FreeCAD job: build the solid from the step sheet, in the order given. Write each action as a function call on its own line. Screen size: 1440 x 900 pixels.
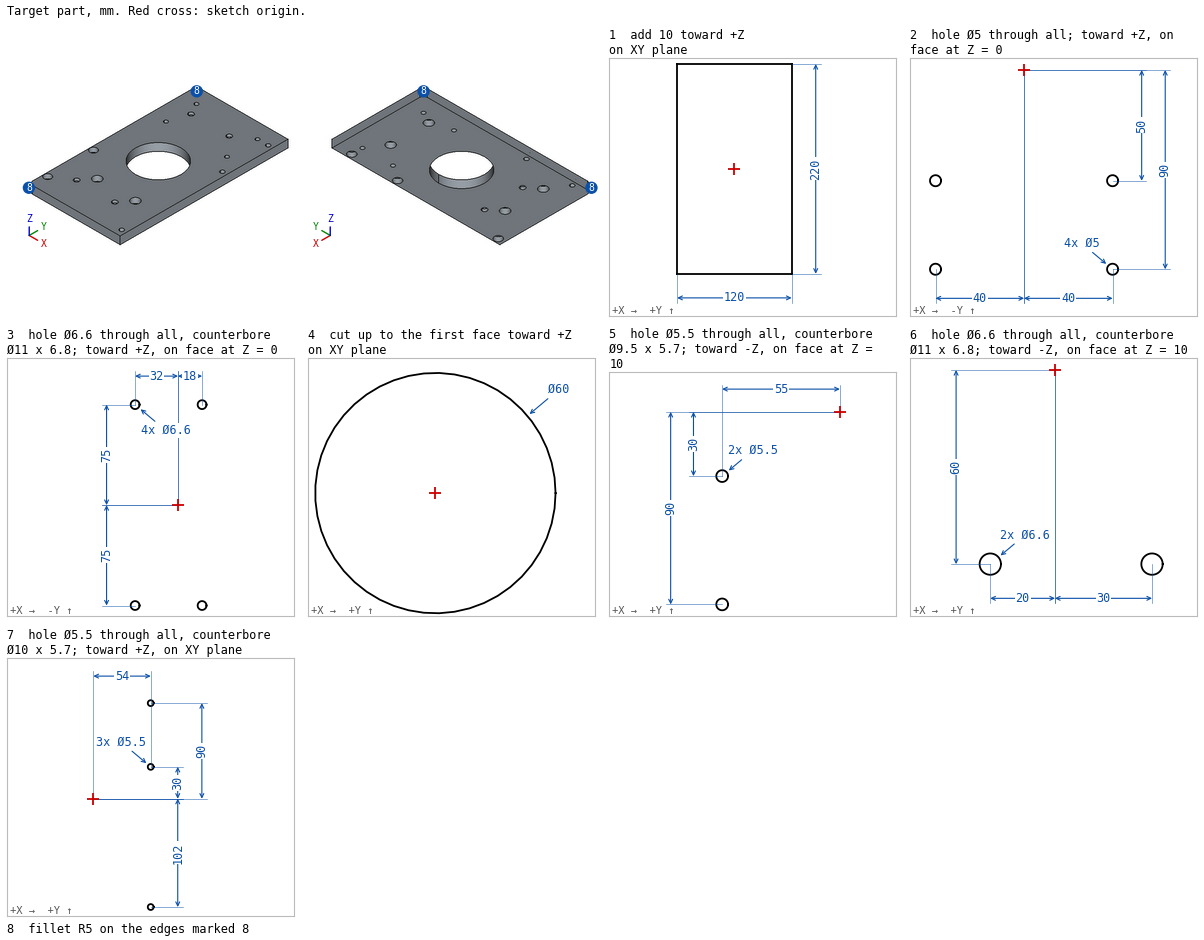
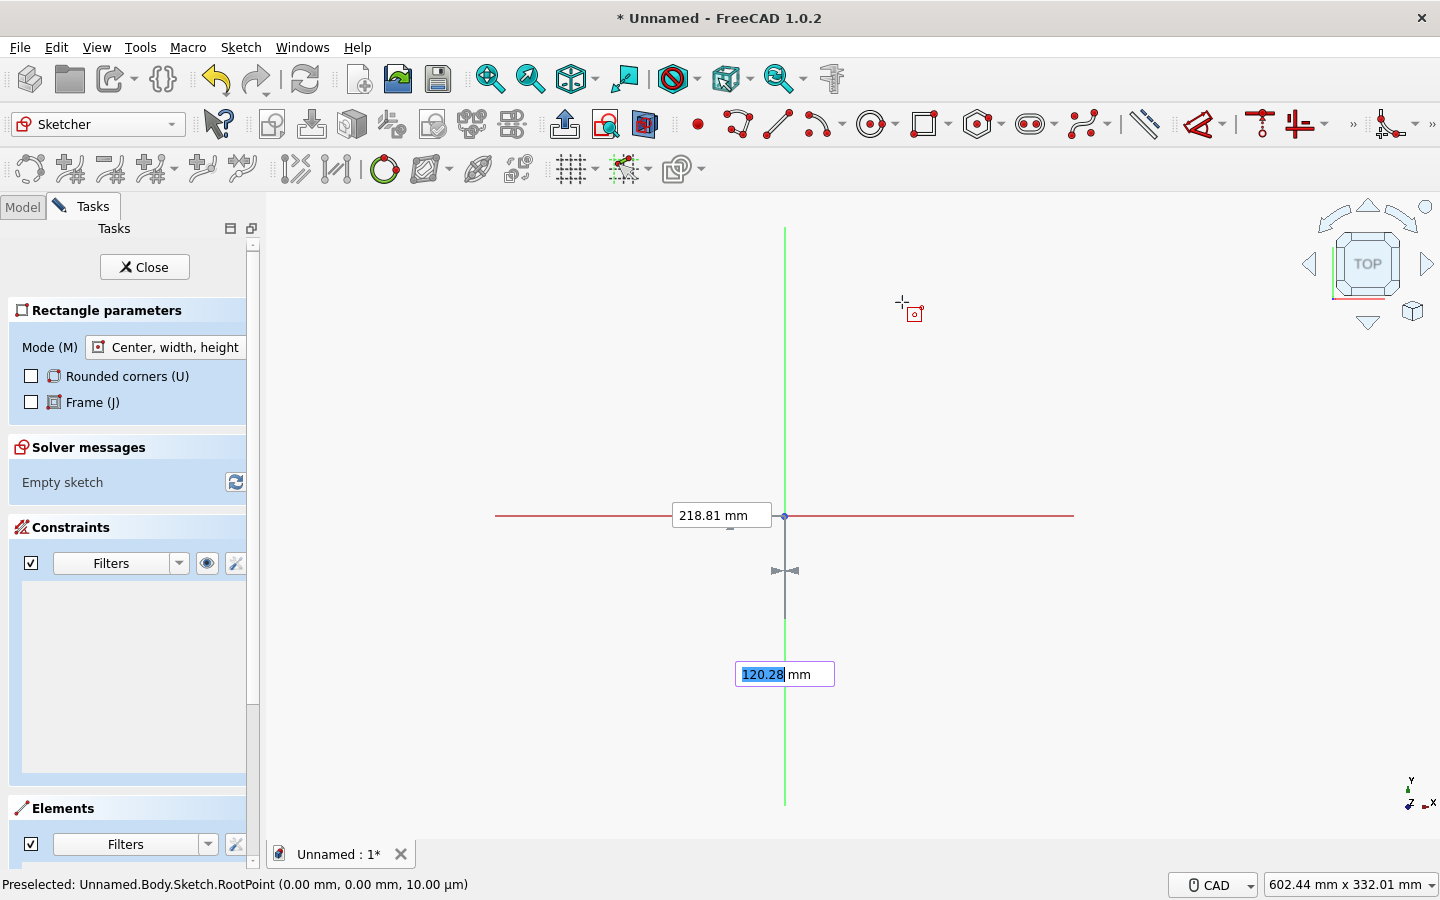
text(120)
key(Tab)
text(220)
key(Return)
key(Escape)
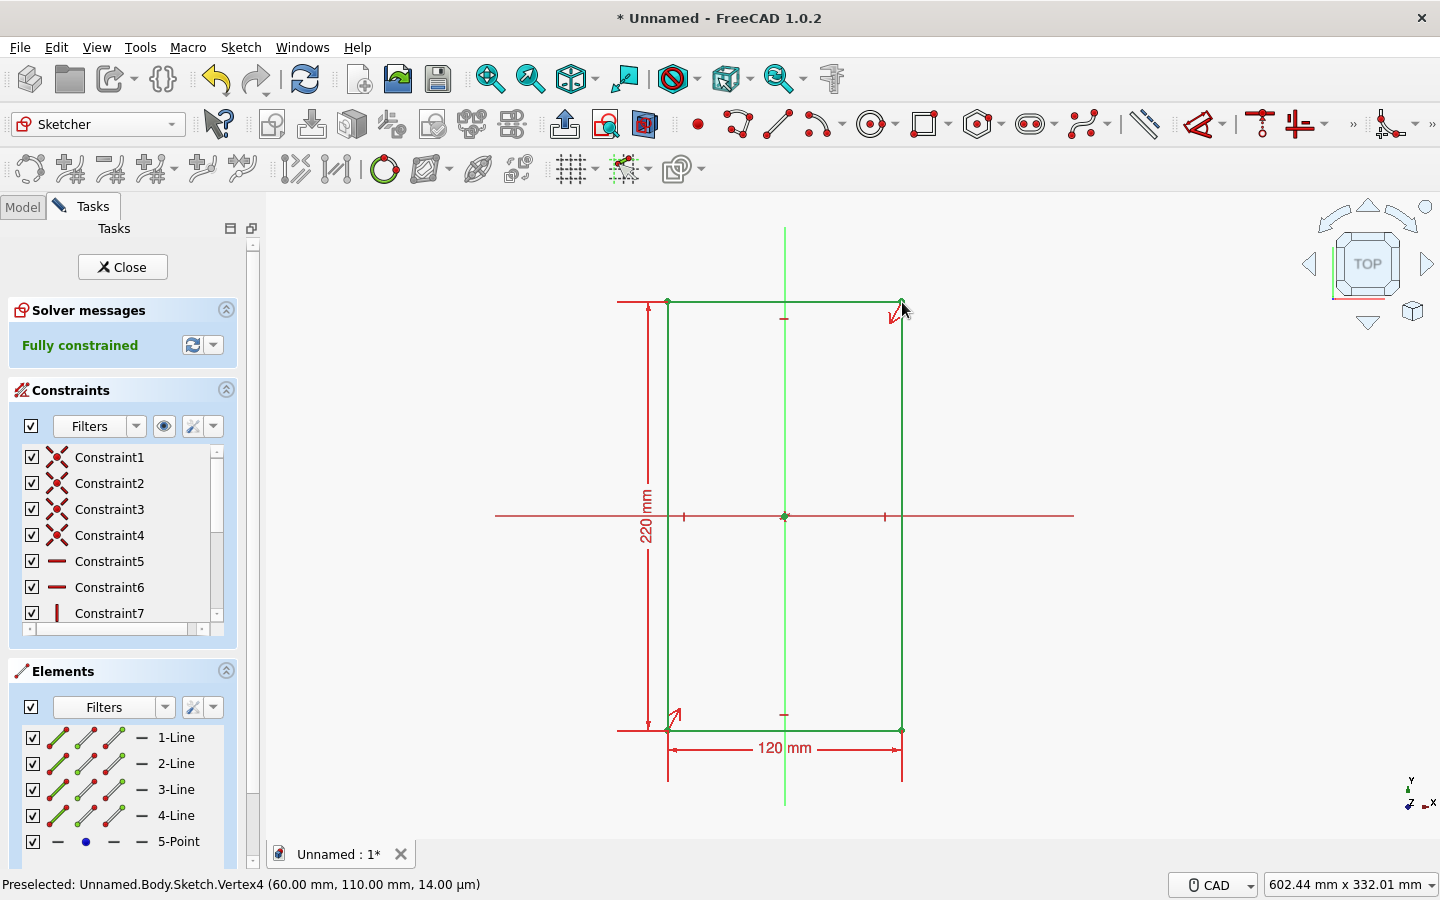
click(123, 267)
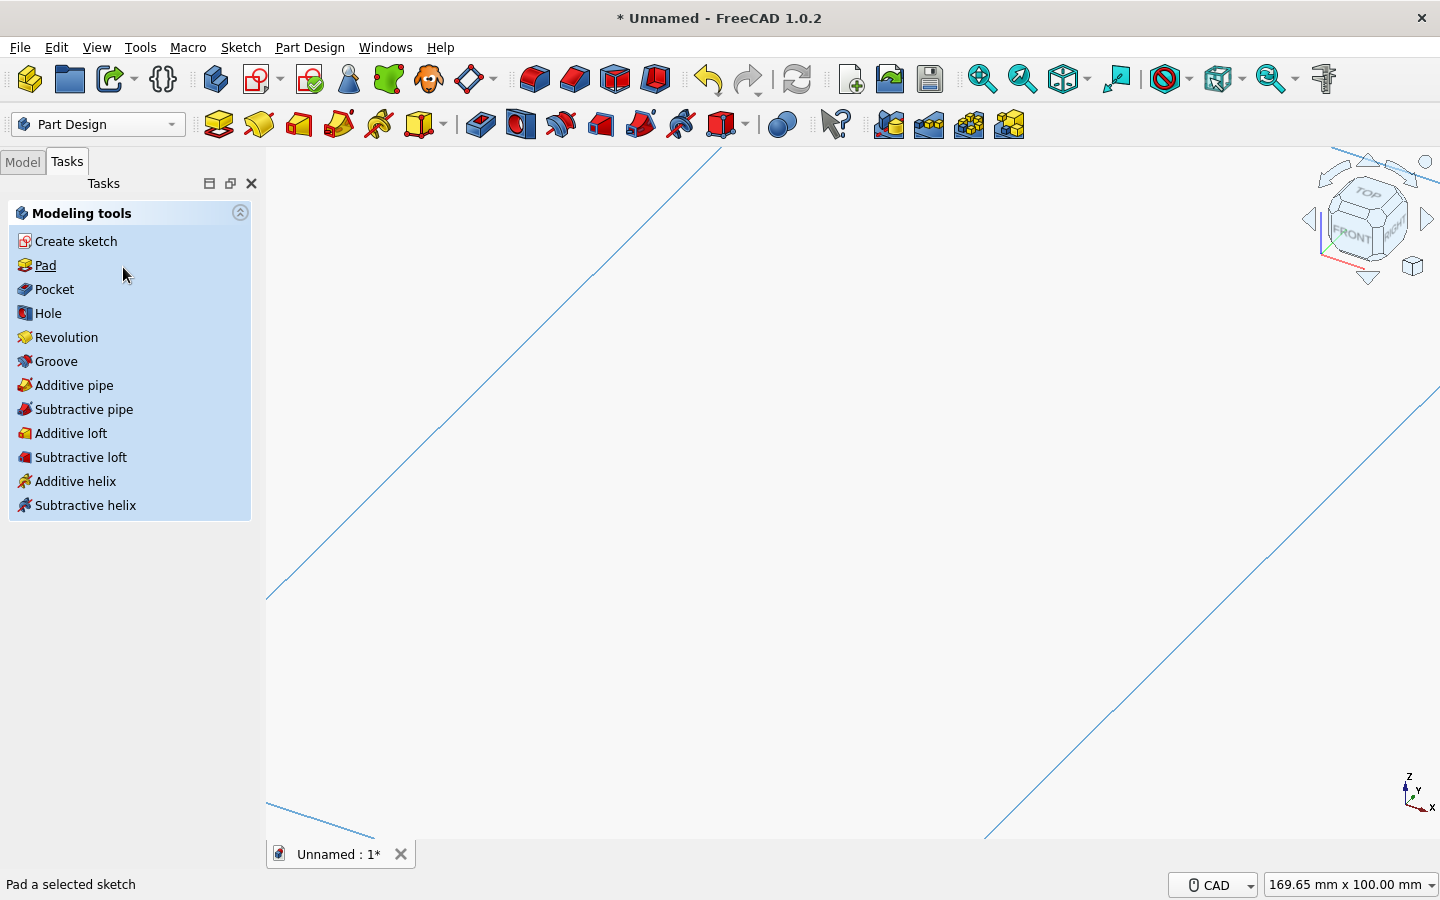
click(220, 124)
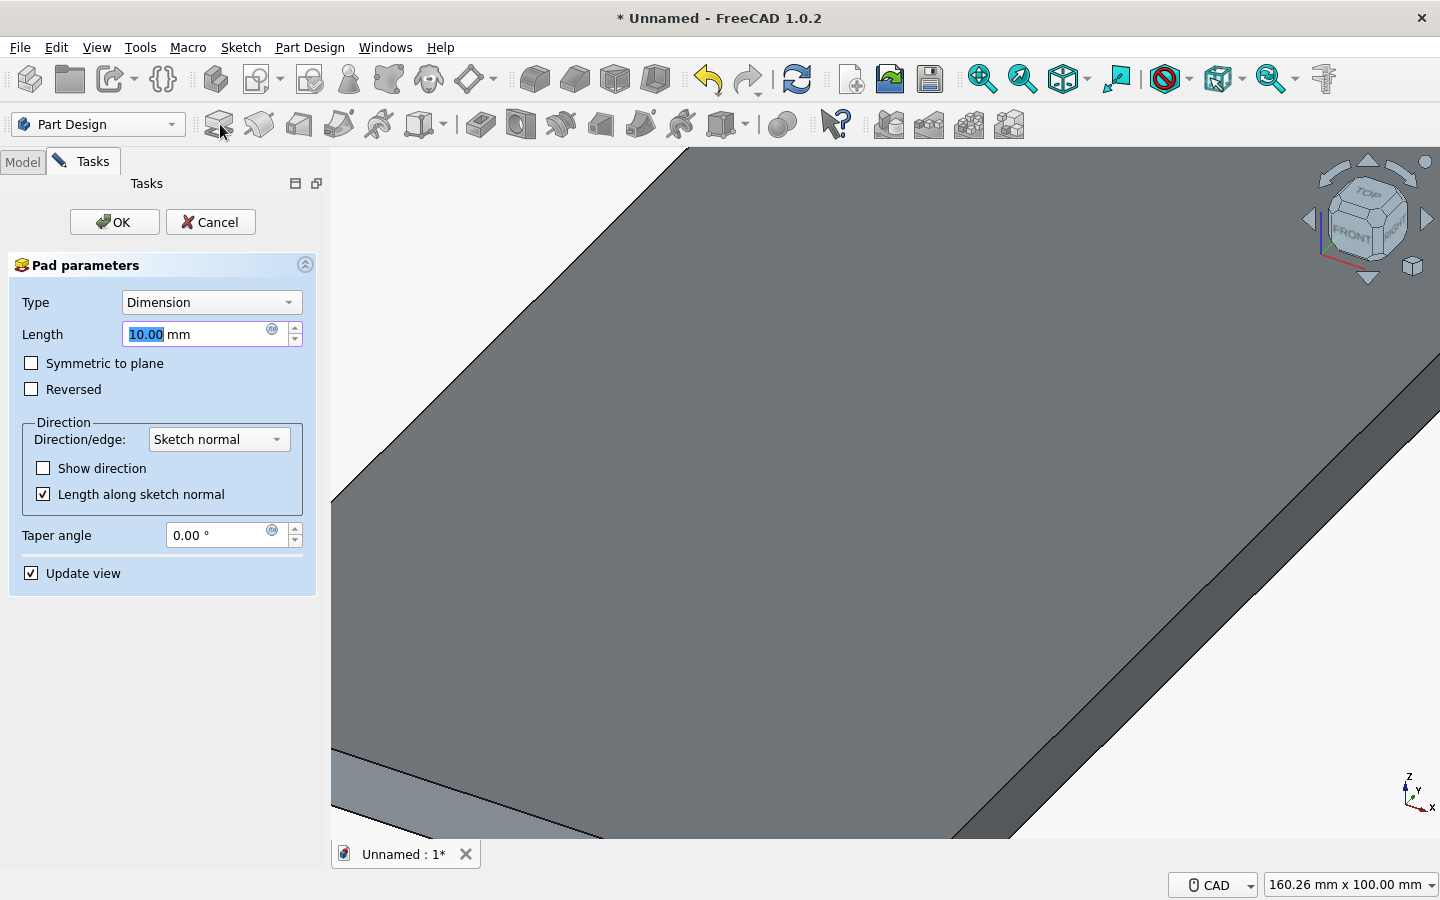
text(10)
key(Tab)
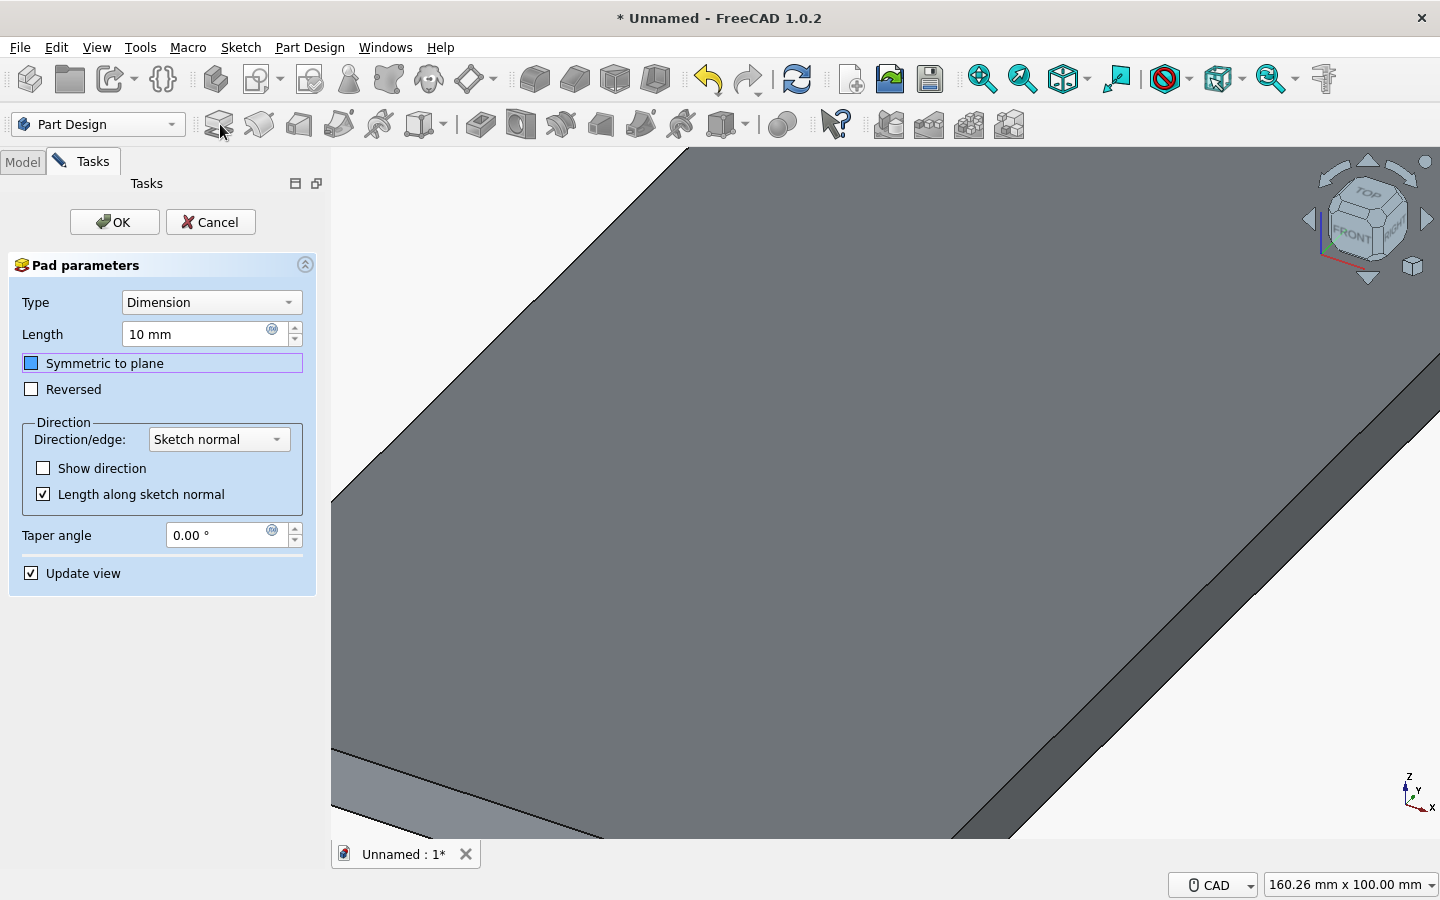
click(115, 222)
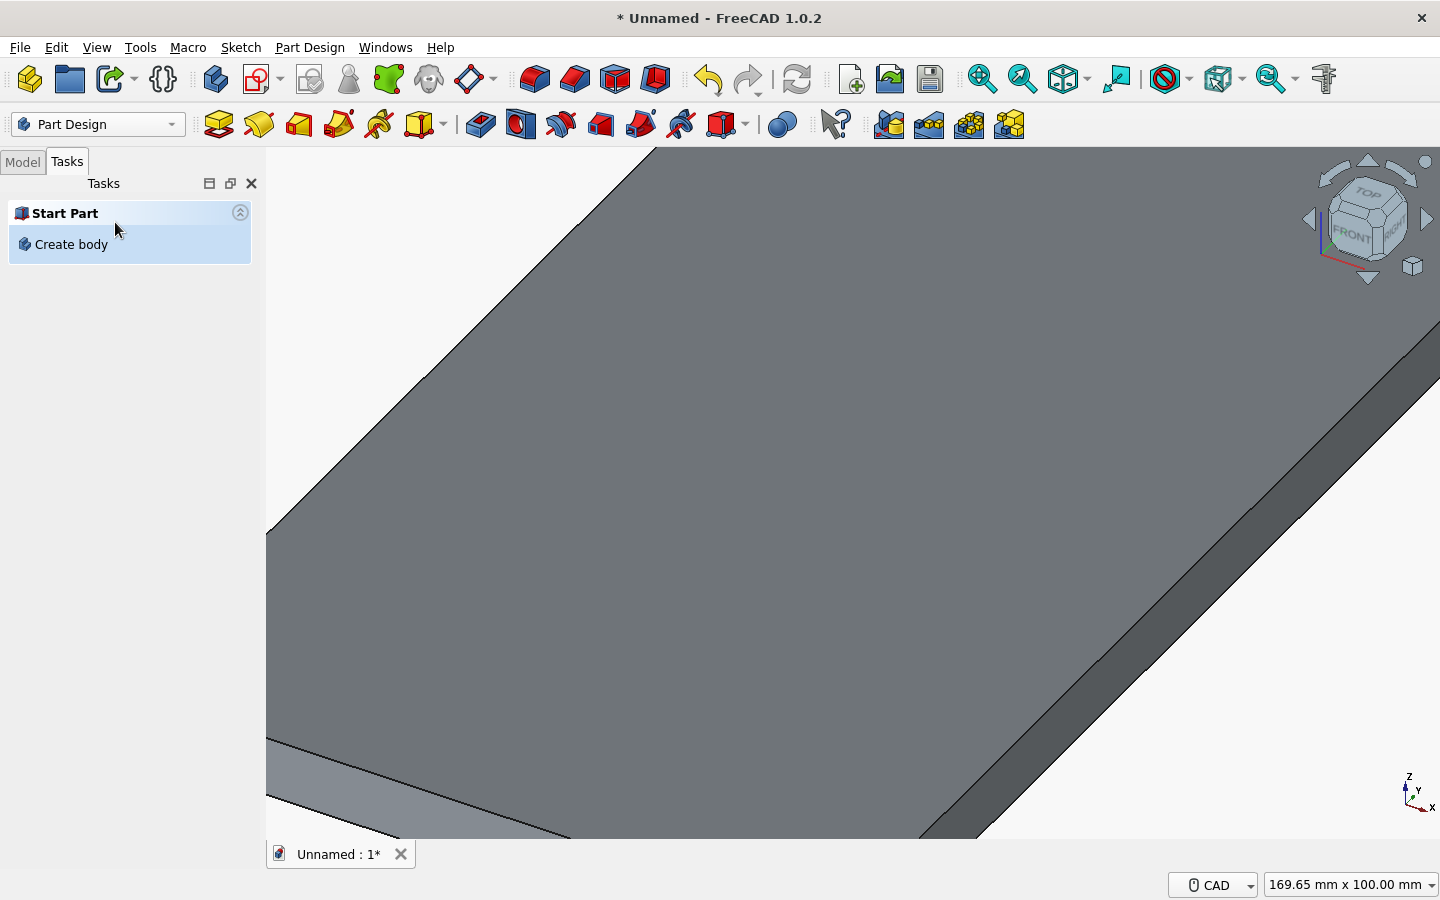
key(v)
key(f)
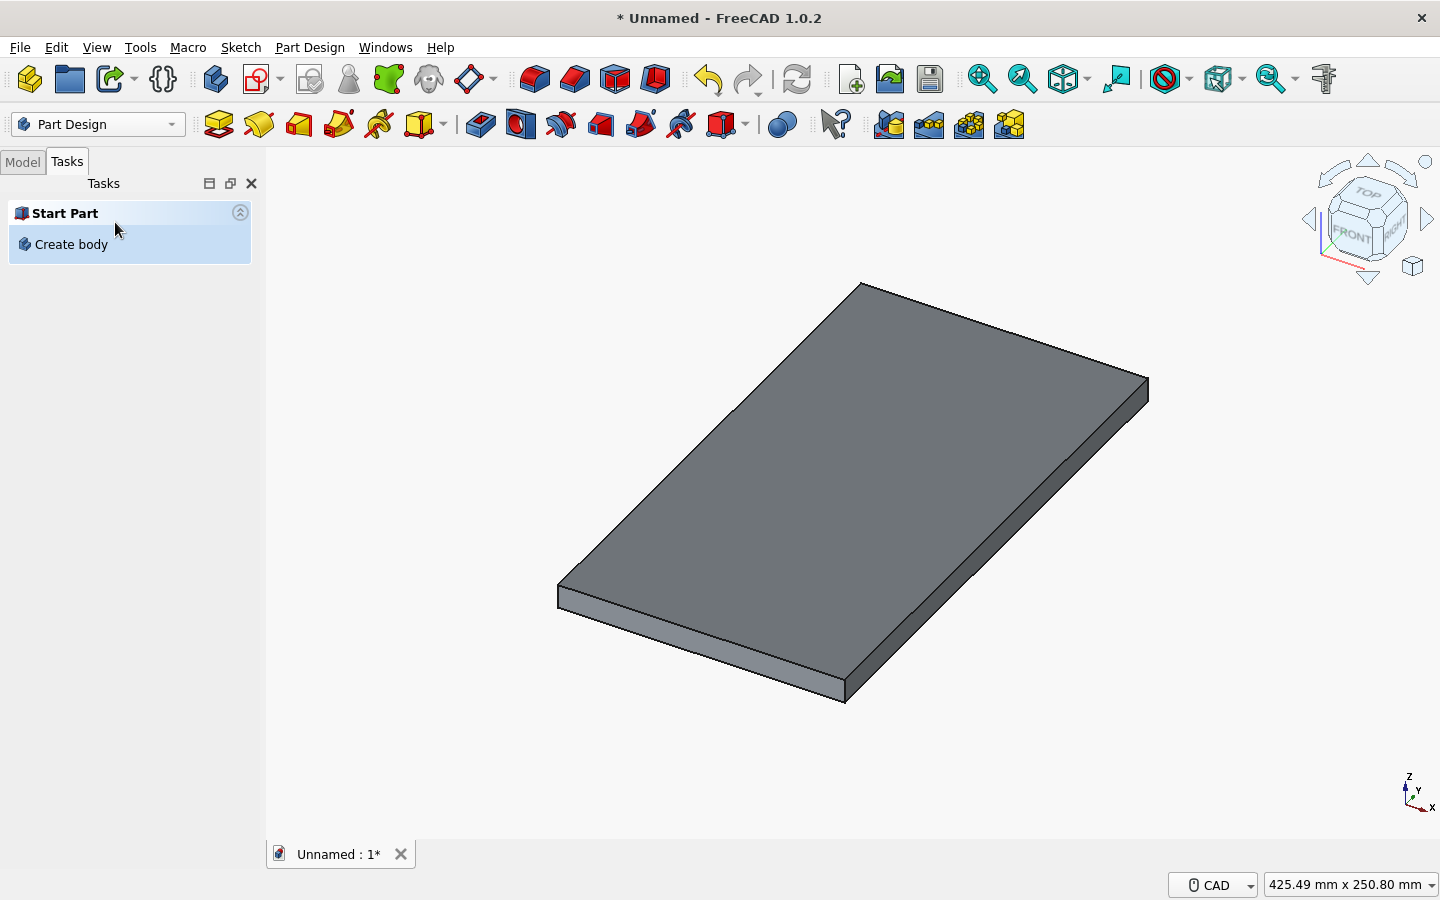
key(5)